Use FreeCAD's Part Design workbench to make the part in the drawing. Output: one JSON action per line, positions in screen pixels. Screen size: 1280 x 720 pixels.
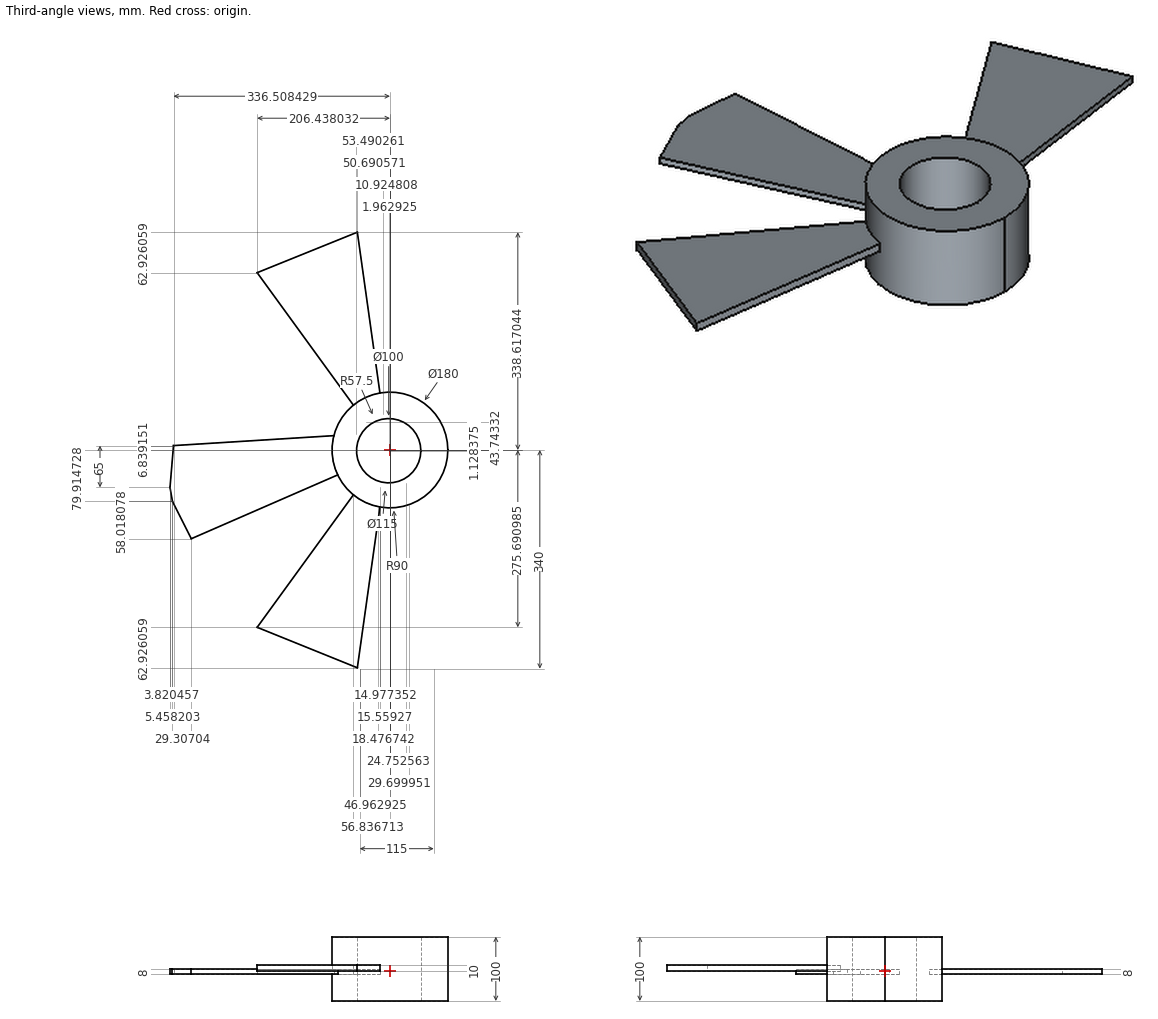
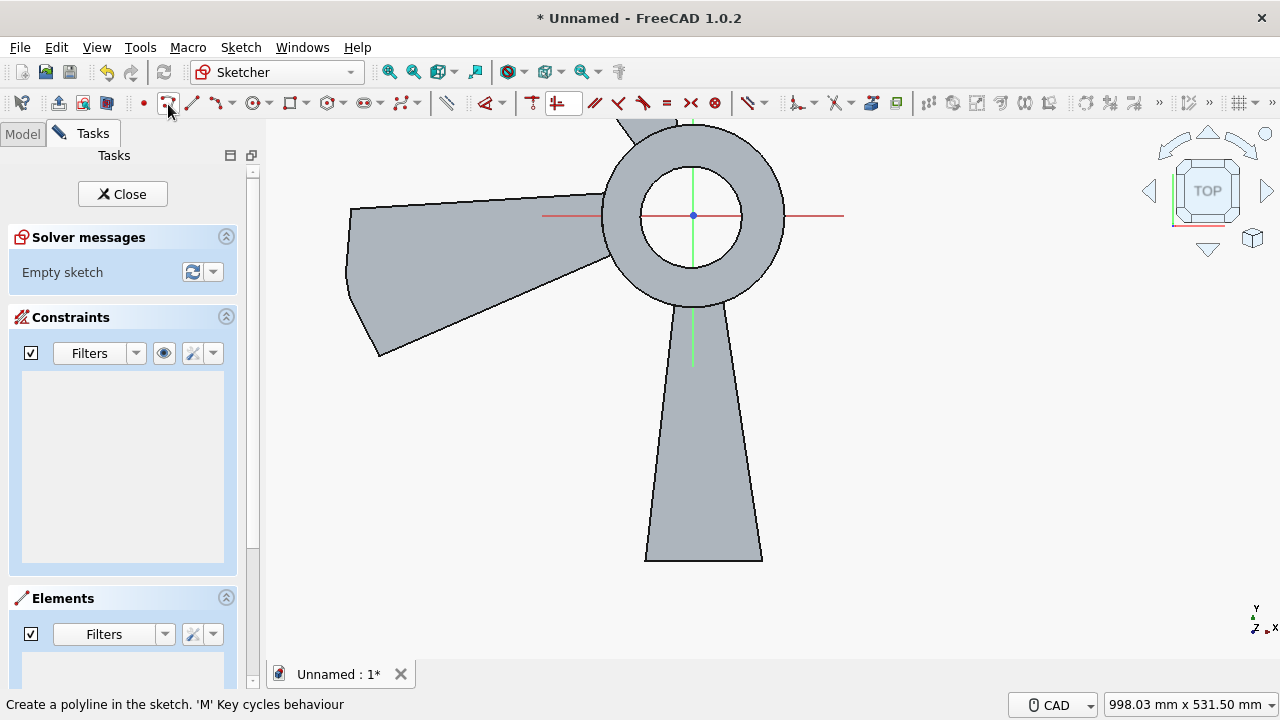
{"action": "left_click", "coordinate": [674, 305]}
{"action": "left_click", "coordinate": [645, 561]}
{"action": "left_click", "coordinate": [762, 561]}
{"action": "left_click", "coordinate": [723, 302]}
{"action": "right_click", "coordinate": [723, 302]}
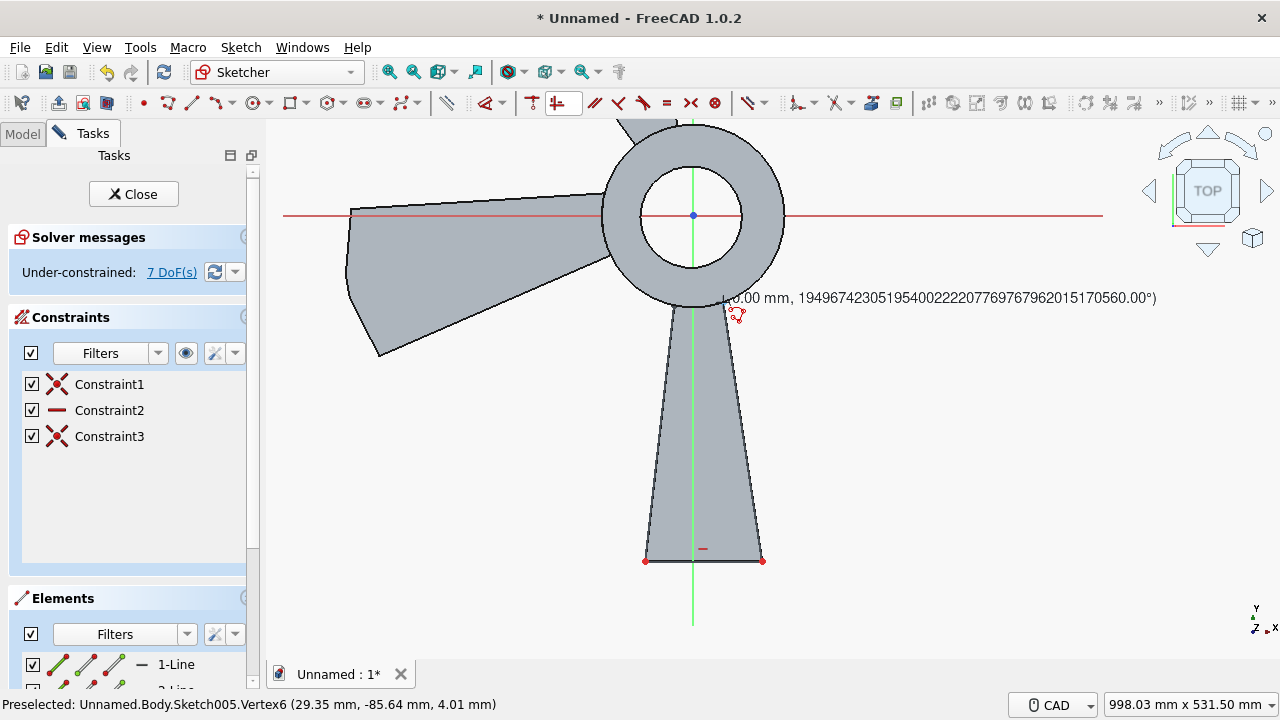
{"action": "left_click", "coordinate": [216, 104]}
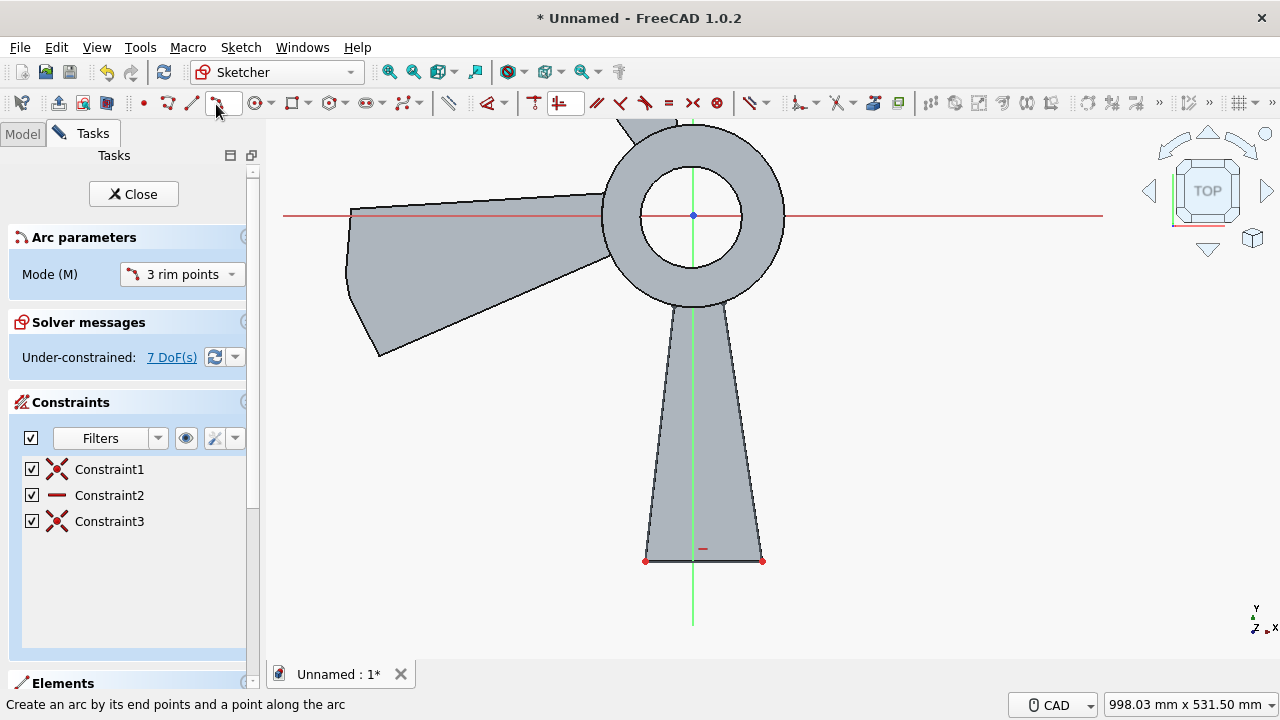
{"action": "left_click", "coordinate": [723, 303]}
{"action": "left_click", "coordinate": [674, 306]}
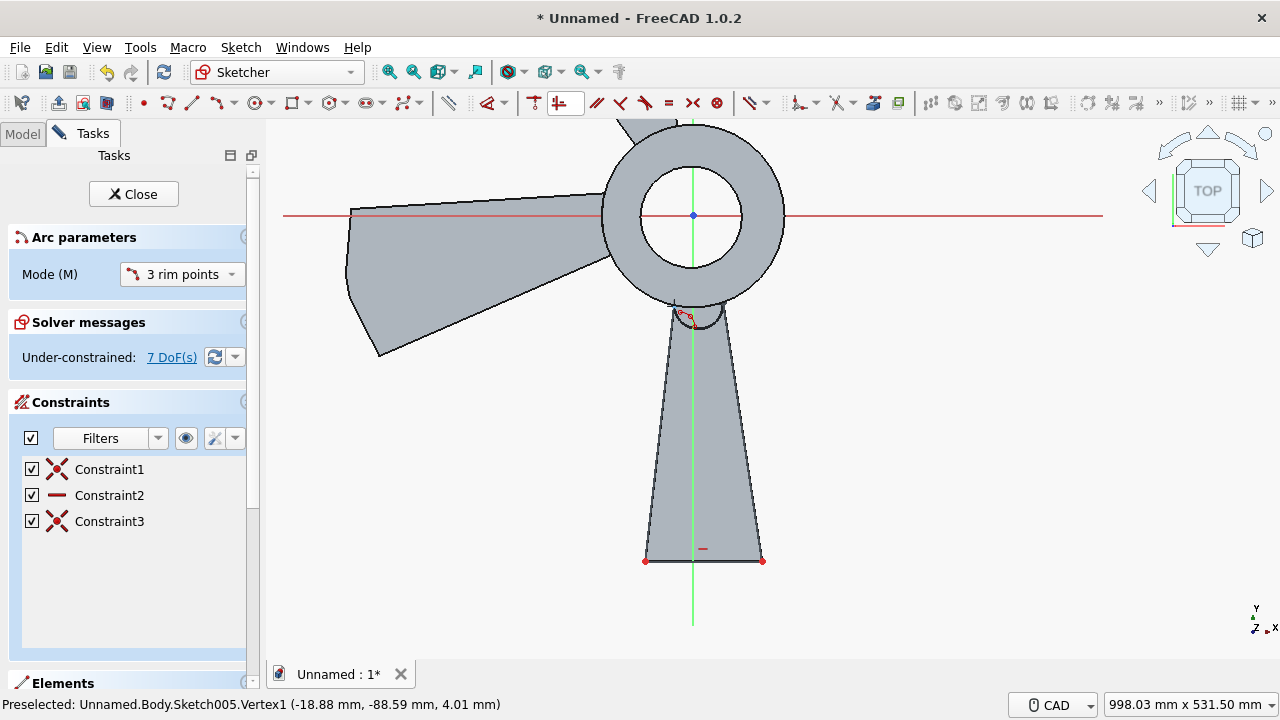
{"action": "scroll", "coordinate": [699, 307], "scroll_direction": "up", "scroll_amount": 8}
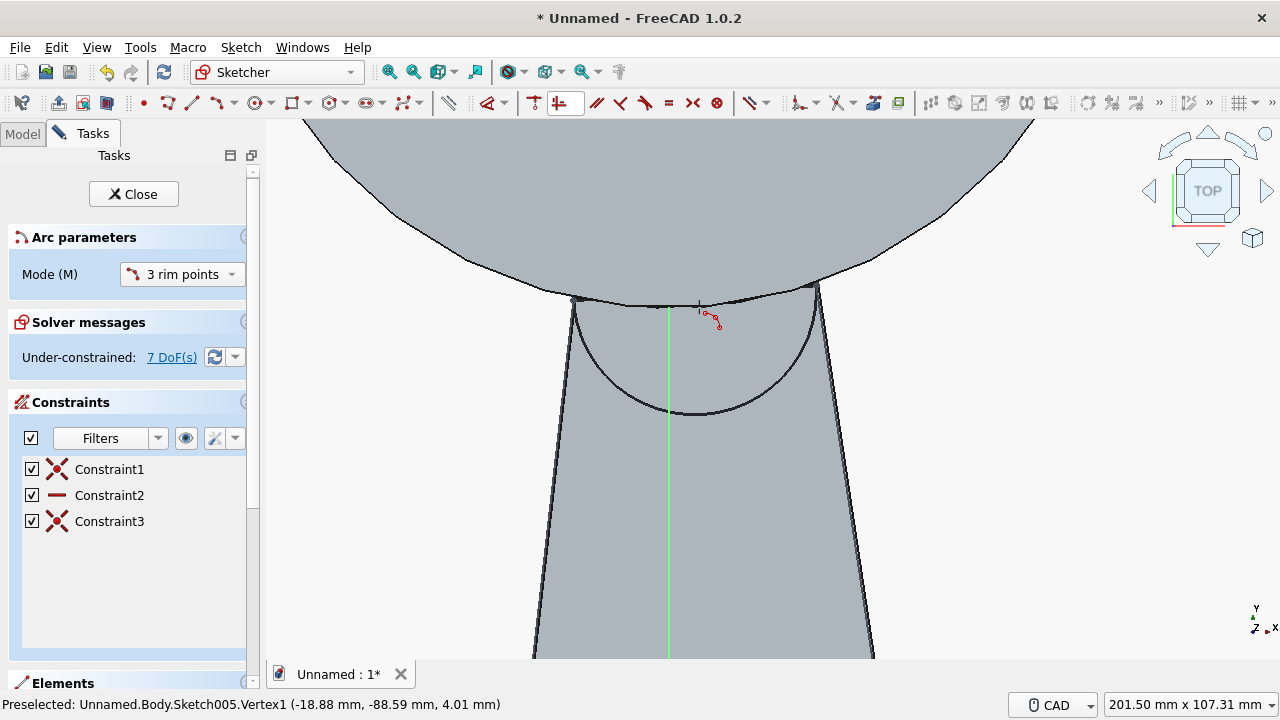
{"action": "left_click", "coordinate": [698, 307]}
{"action": "key", "text": "Escape"}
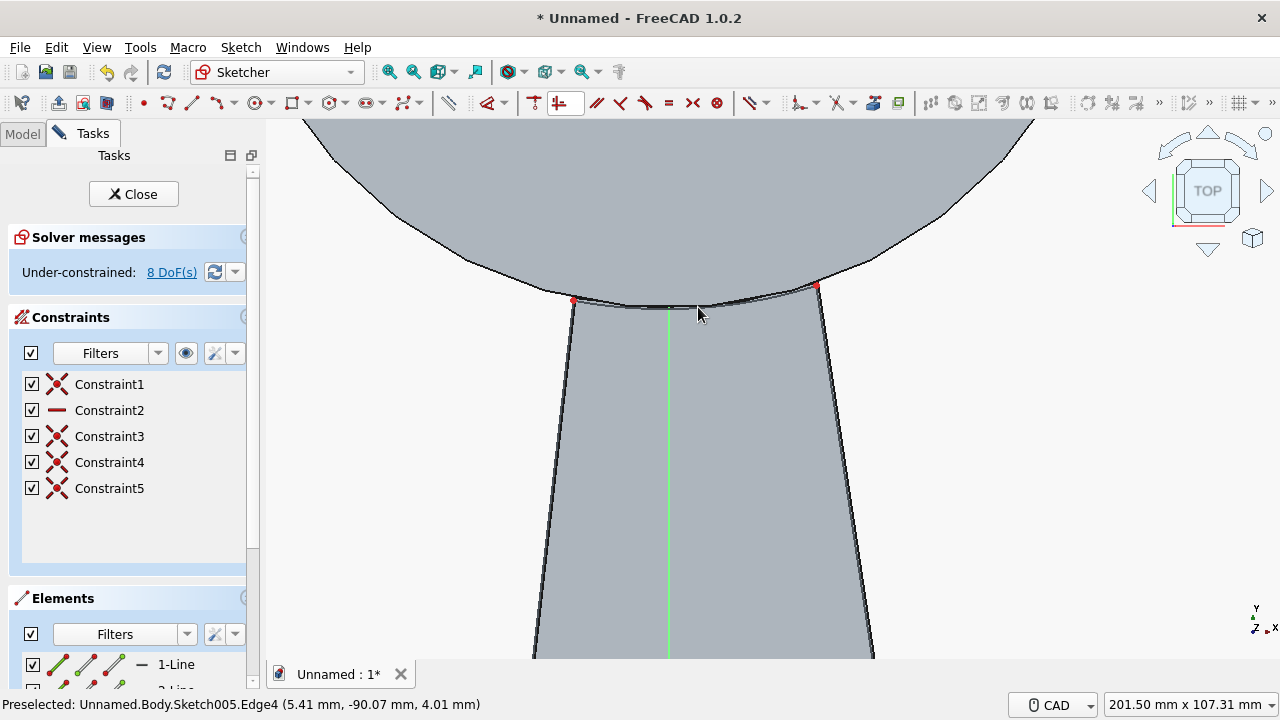
{"action": "scroll", "coordinate": [700, 308], "scroll_direction": "down", "scroll_amount": 8}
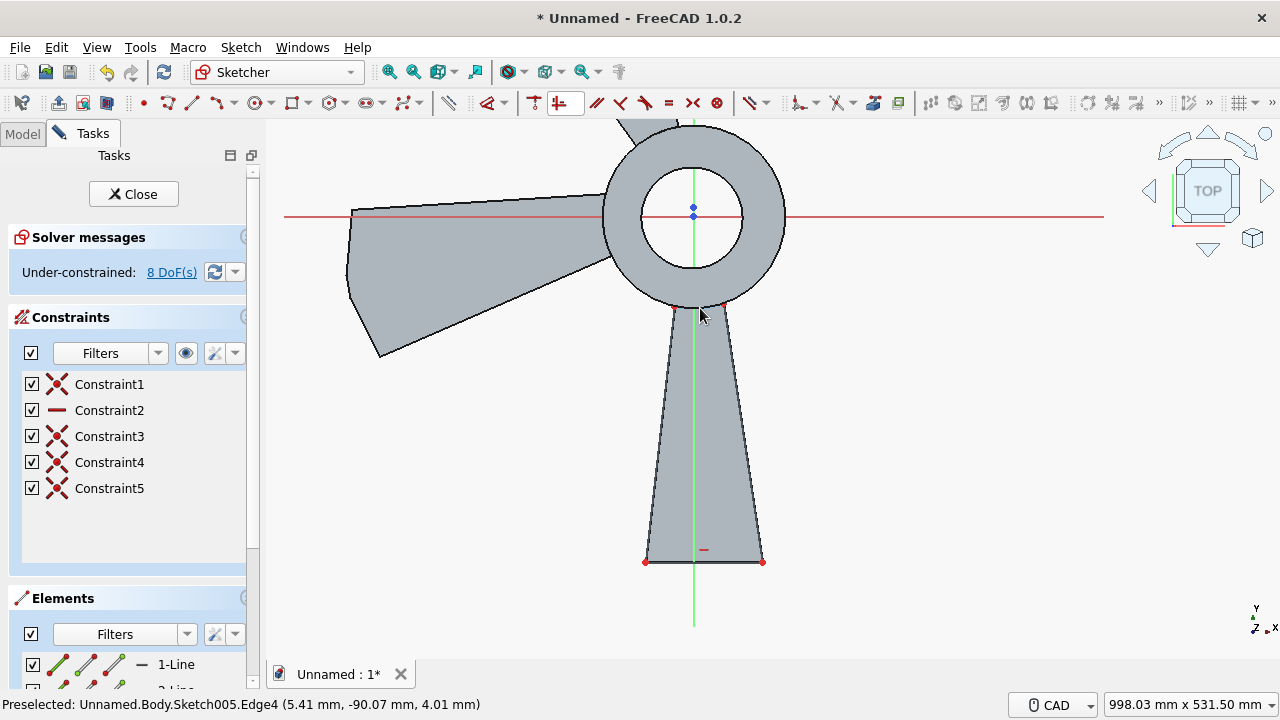
{"action": "left_click_drag", "start_coordinate": [683, 197], "coordinate": [704, 227]}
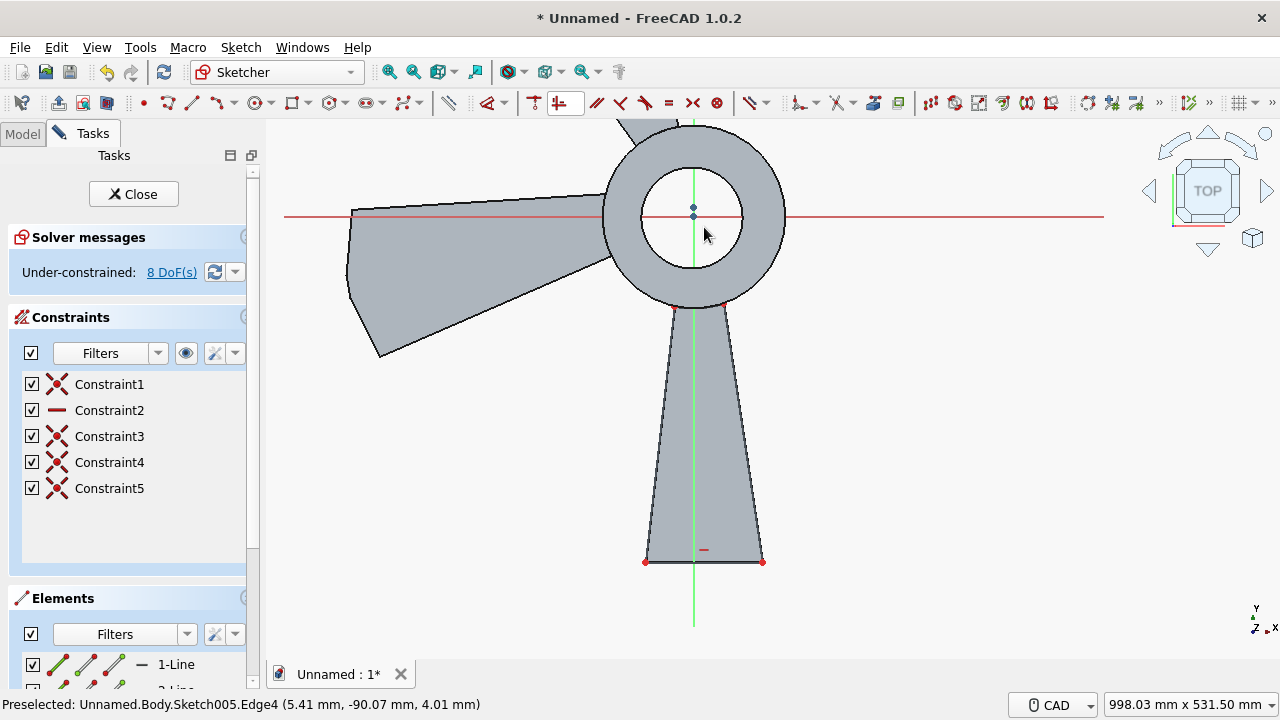
{"action": "left_click", "coordinate": [534, 104]}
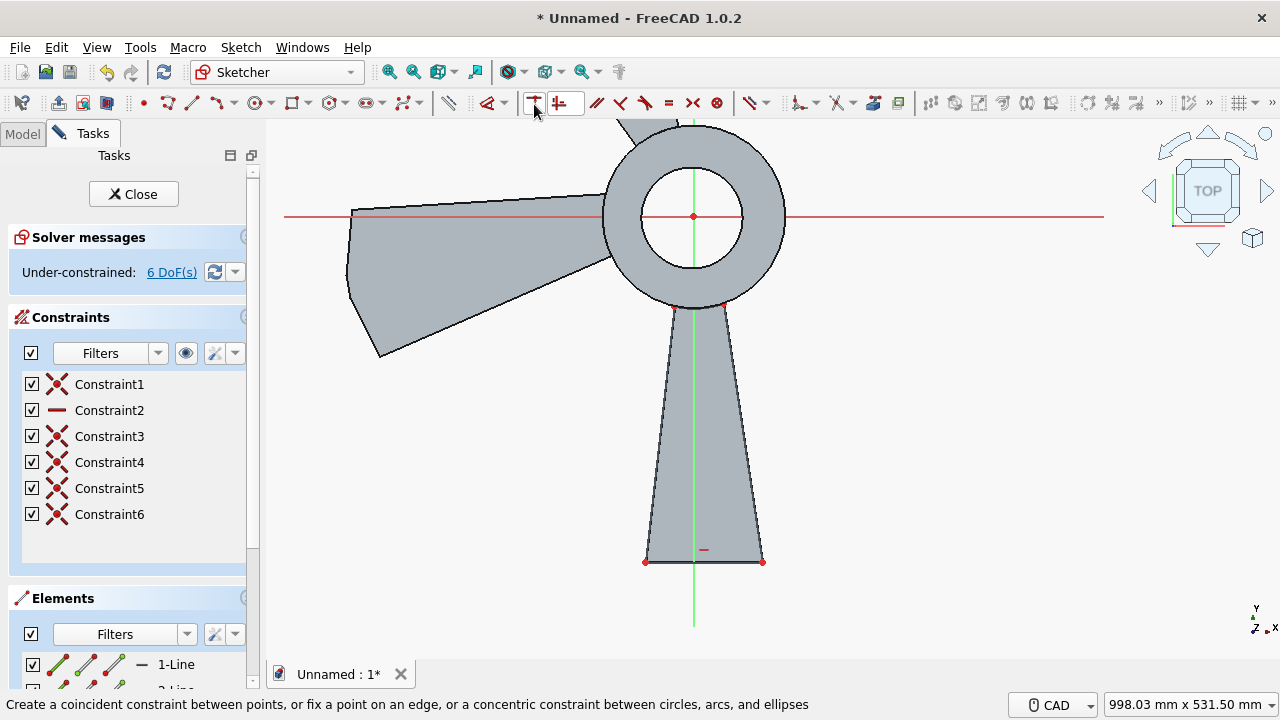
{"action": "left_click", "coordinate": [488, 104]}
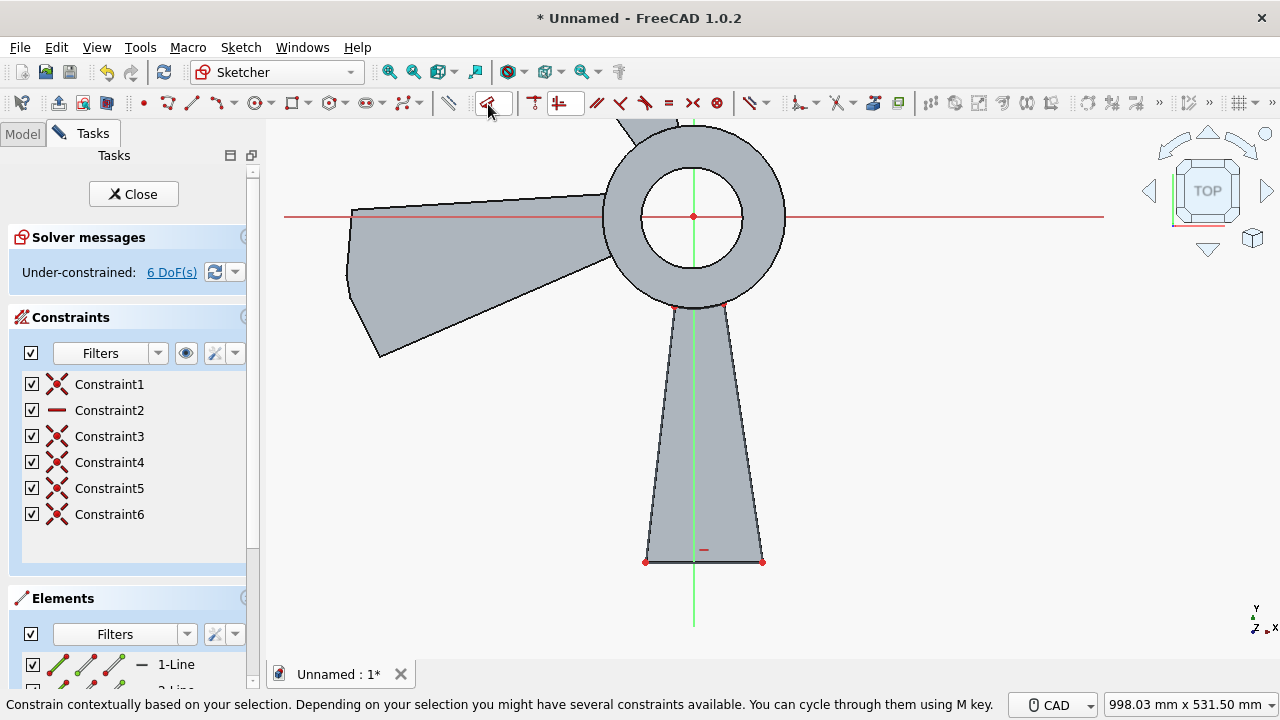
{"action": "left_click", "coordinate": [709, 307]}
{"action": "left_click", "coordinate": [714, 339]}